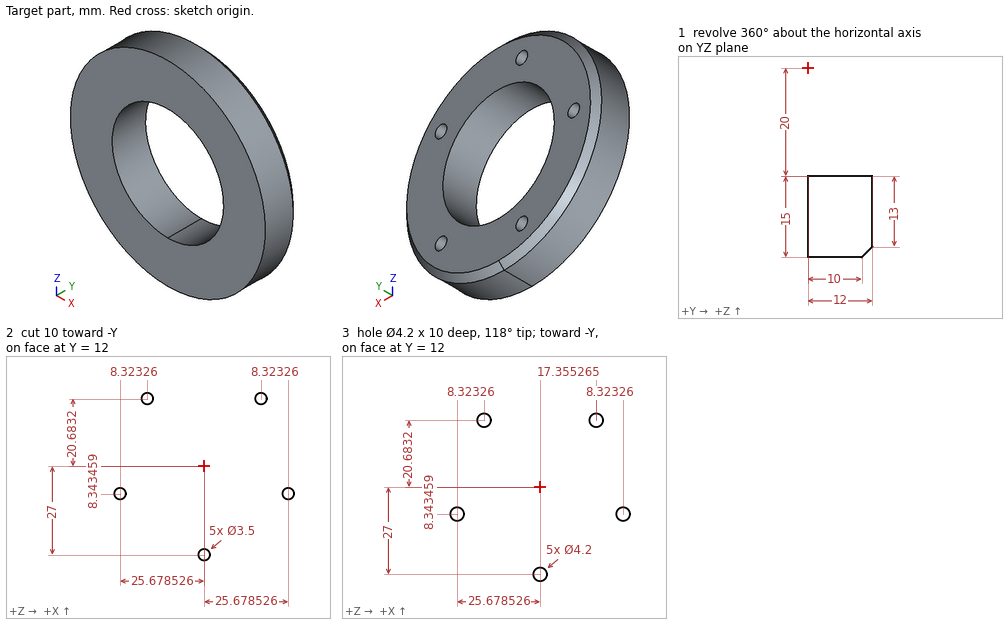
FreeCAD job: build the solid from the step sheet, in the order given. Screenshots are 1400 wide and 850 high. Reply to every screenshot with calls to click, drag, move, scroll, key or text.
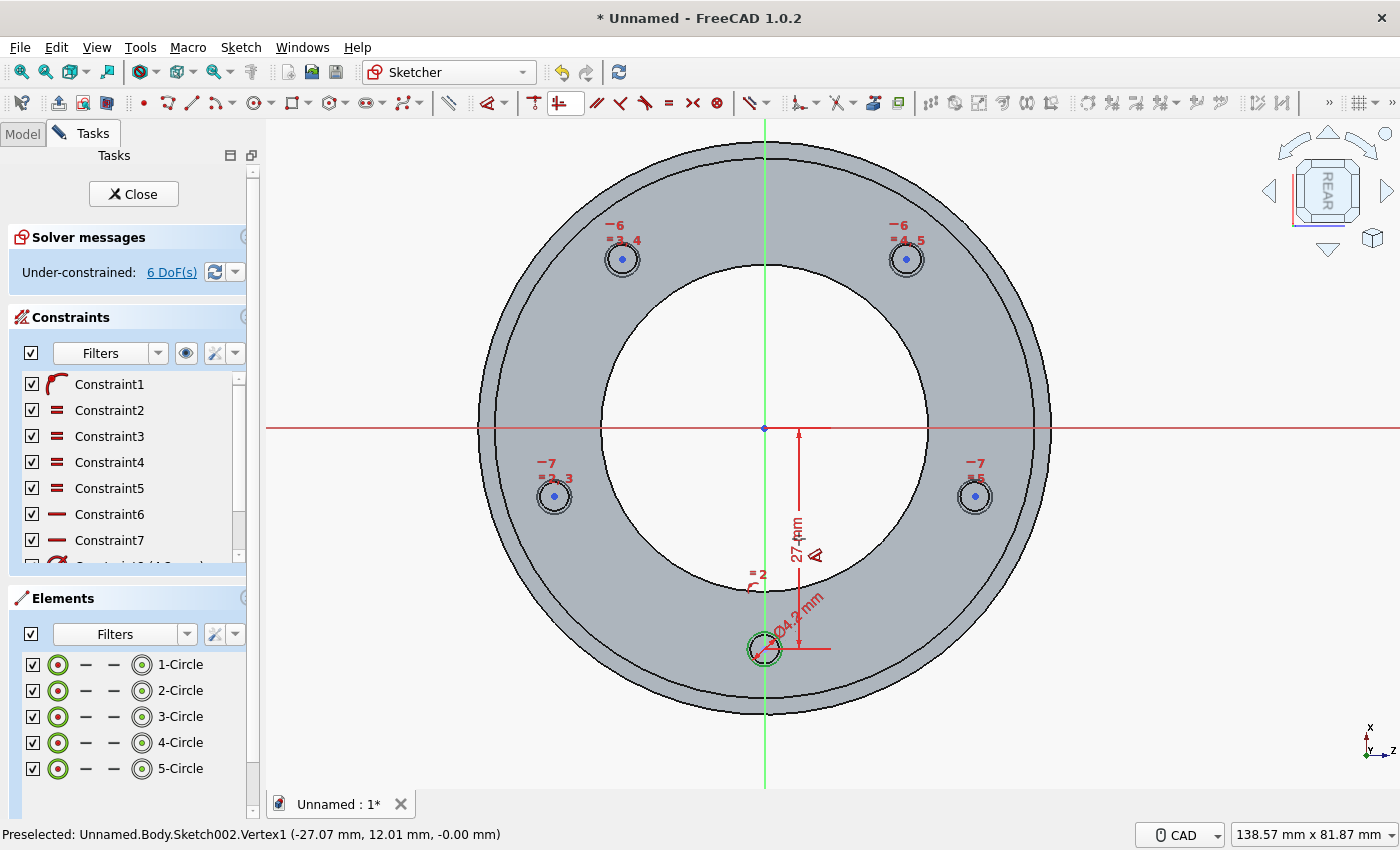
click(622, 260)
click(588, 344)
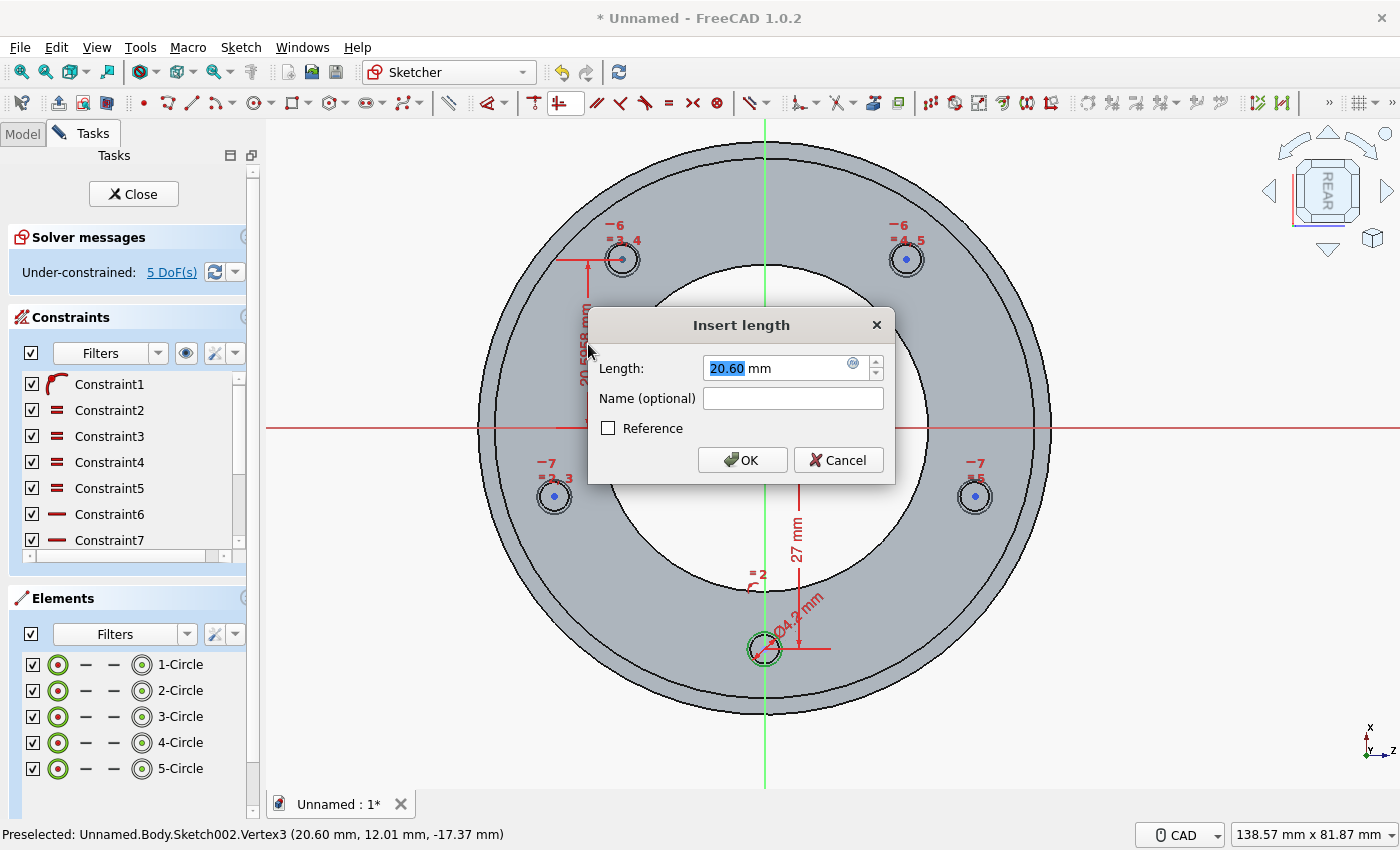
text(20.6832)
key(Return)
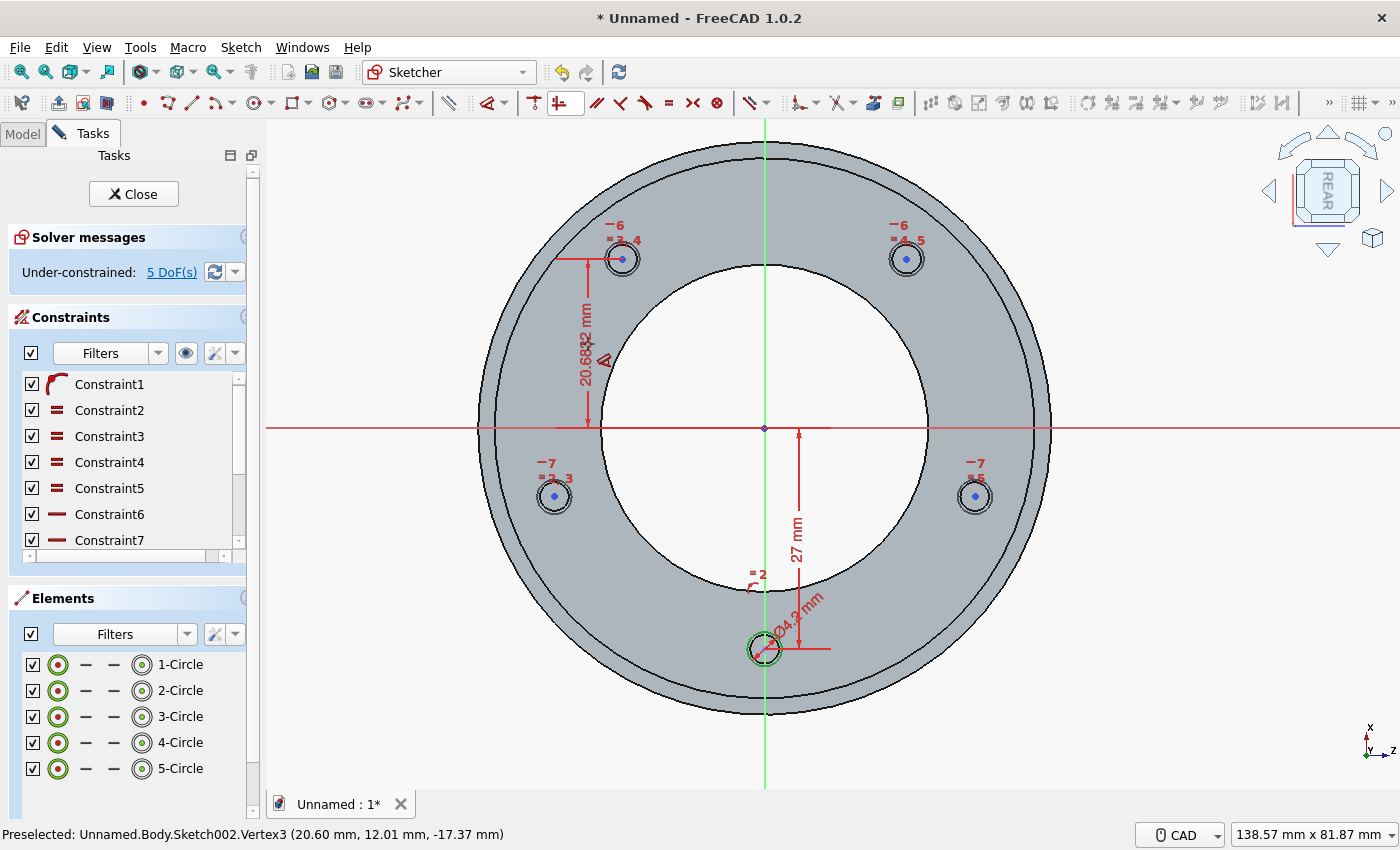
click(554, 497)
click(520, 463)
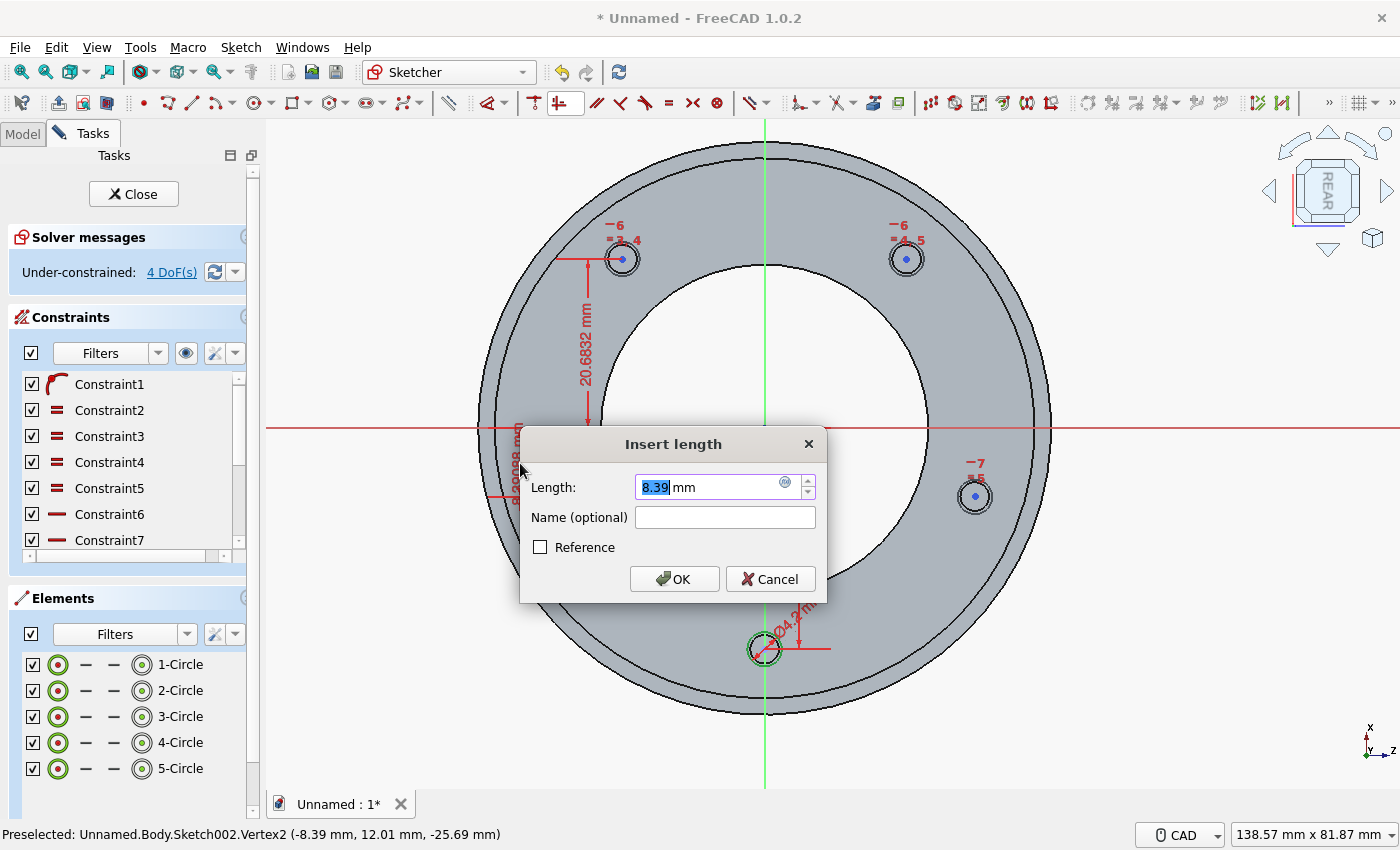
text(8.343459)
key(Return)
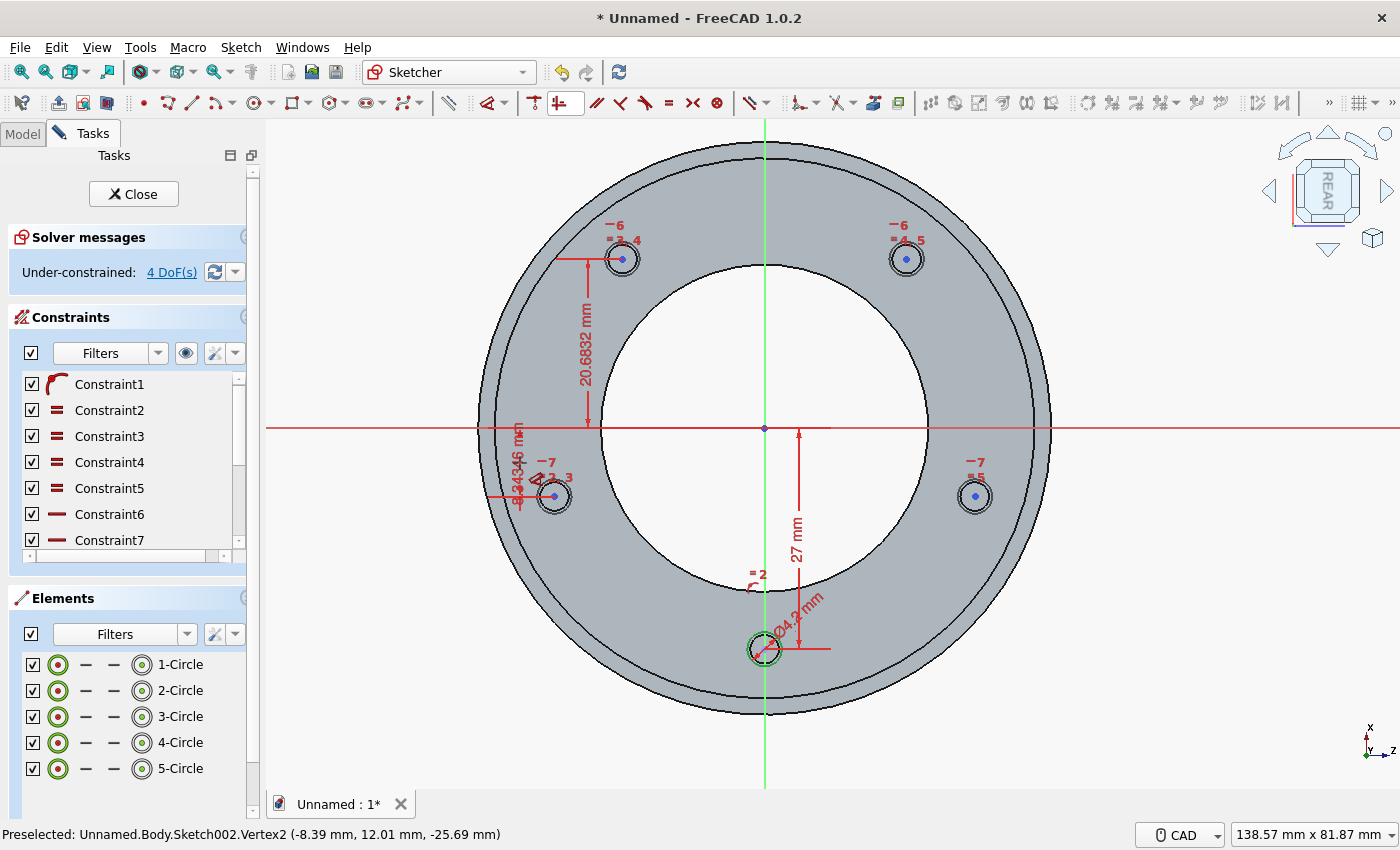
click(554, 497)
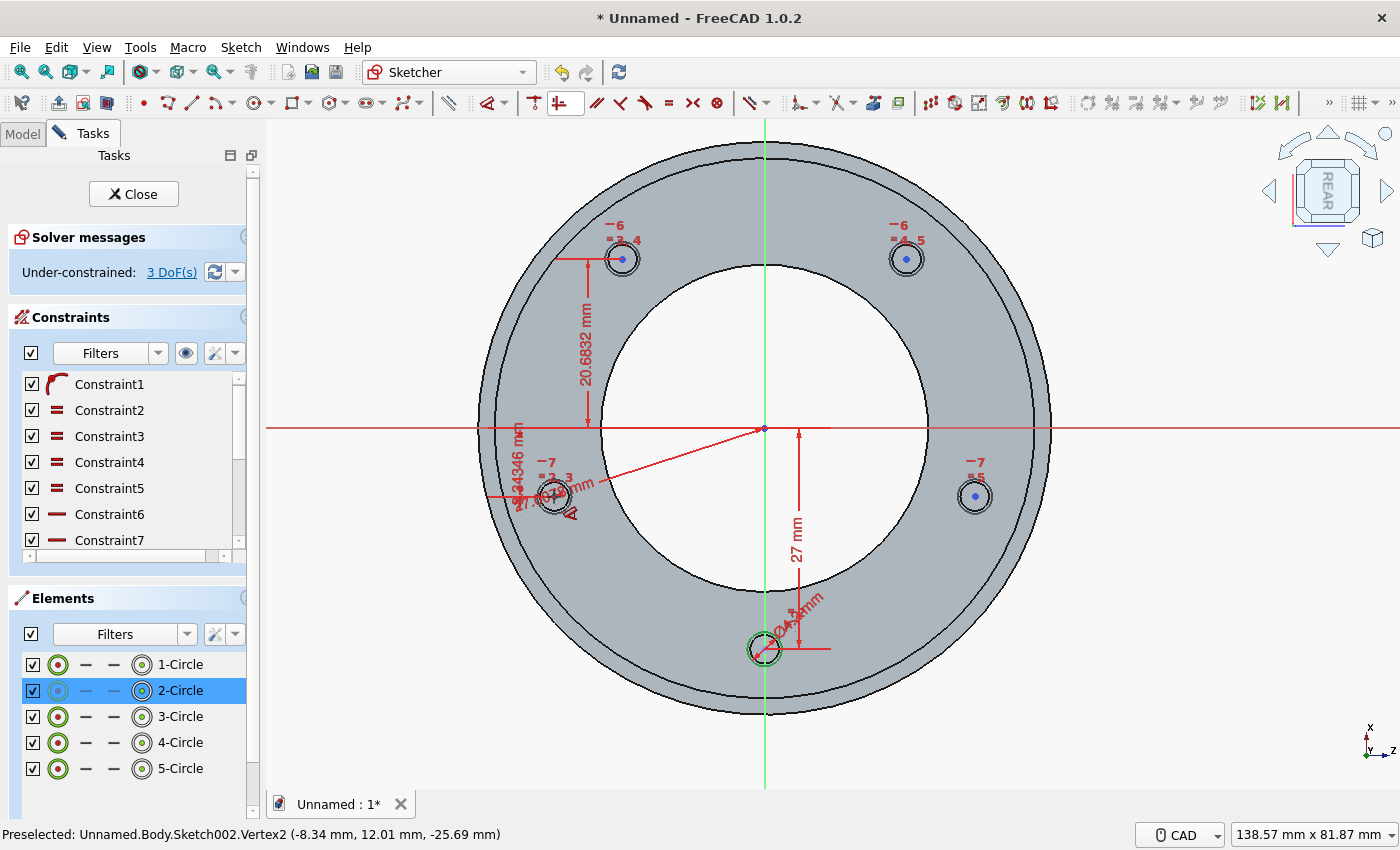
click(622, 259)
click(588, 225)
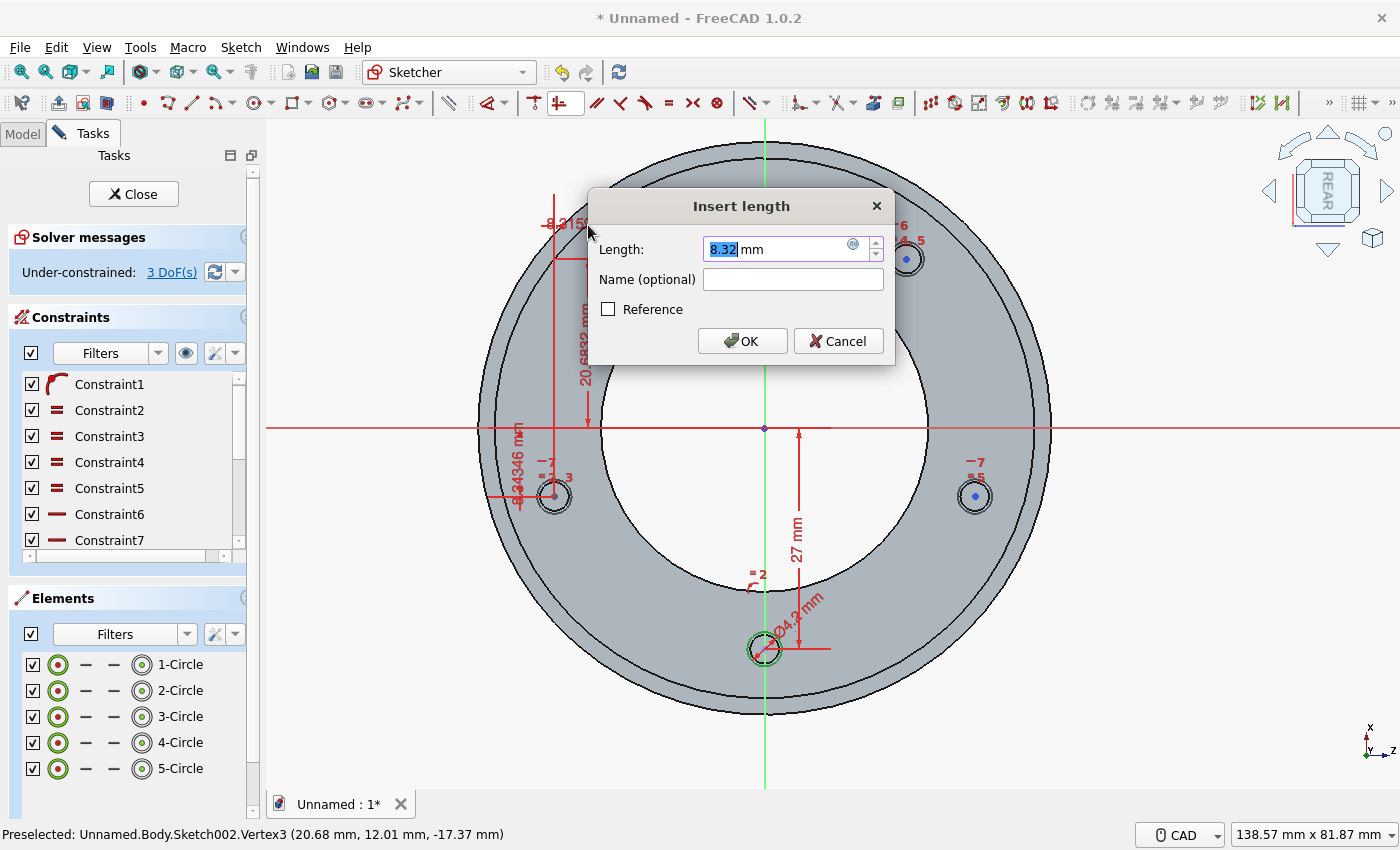
text(8.32326)
key(Return)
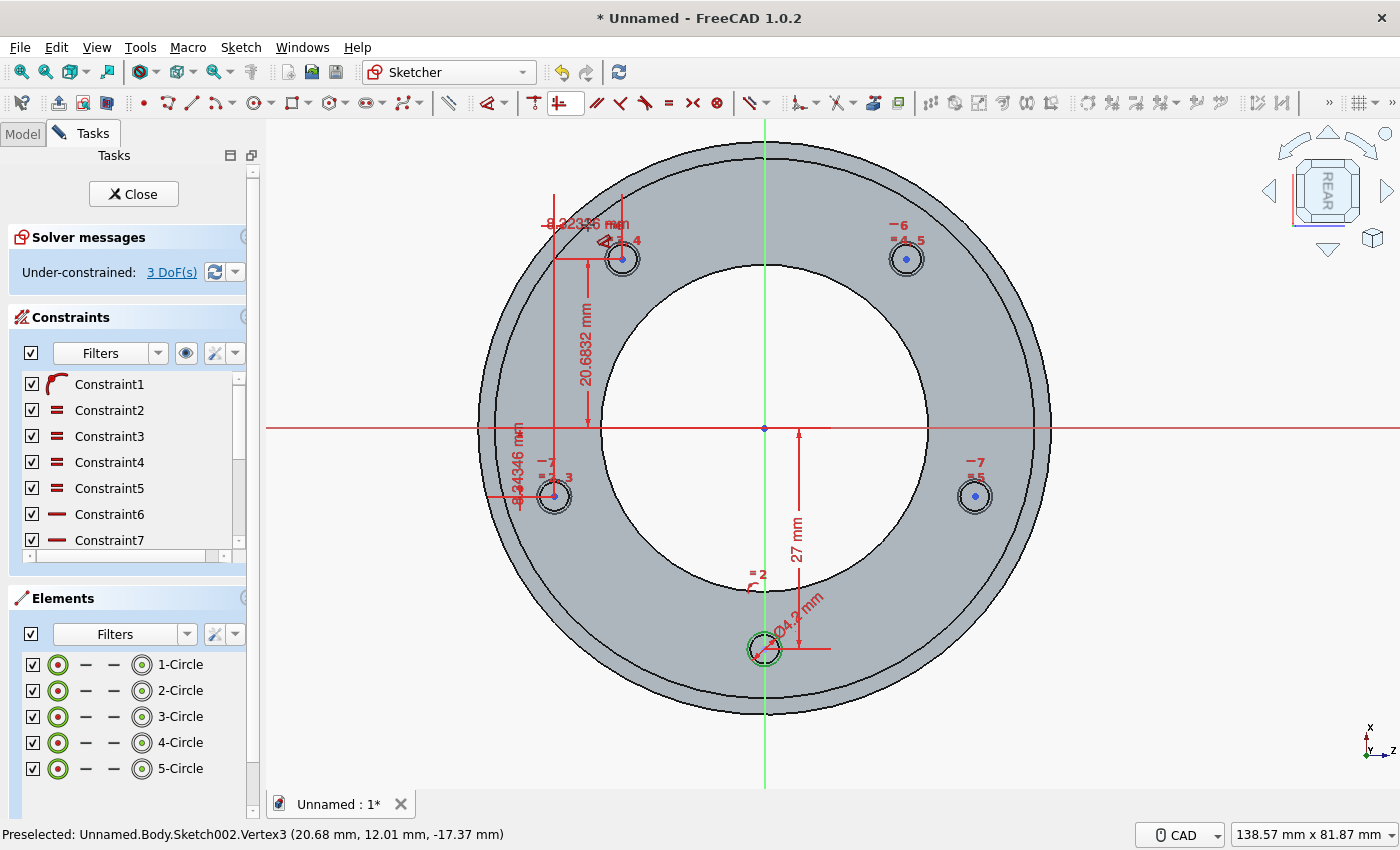
click(907, 259)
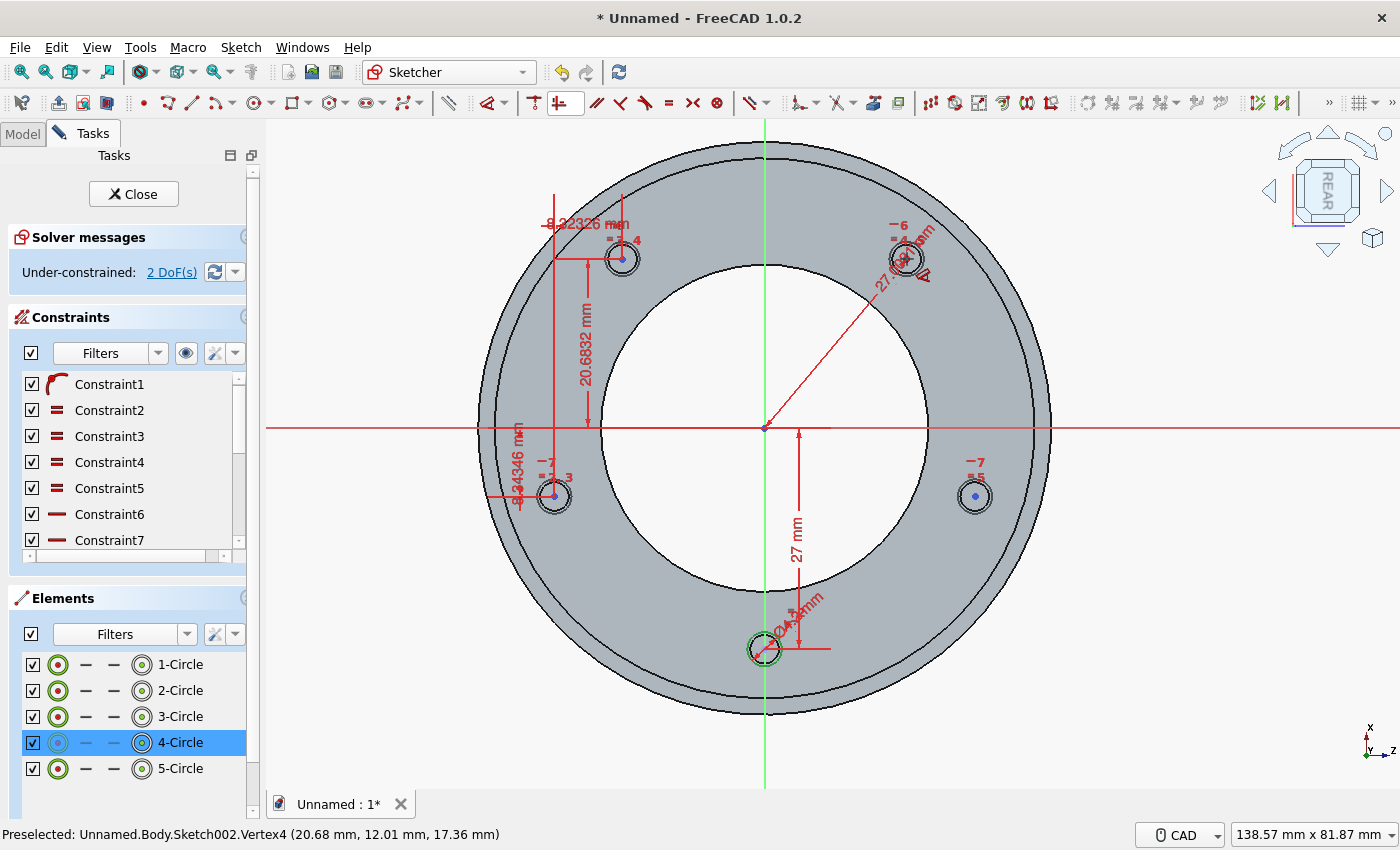
click(975, 497)
click(941, 225)